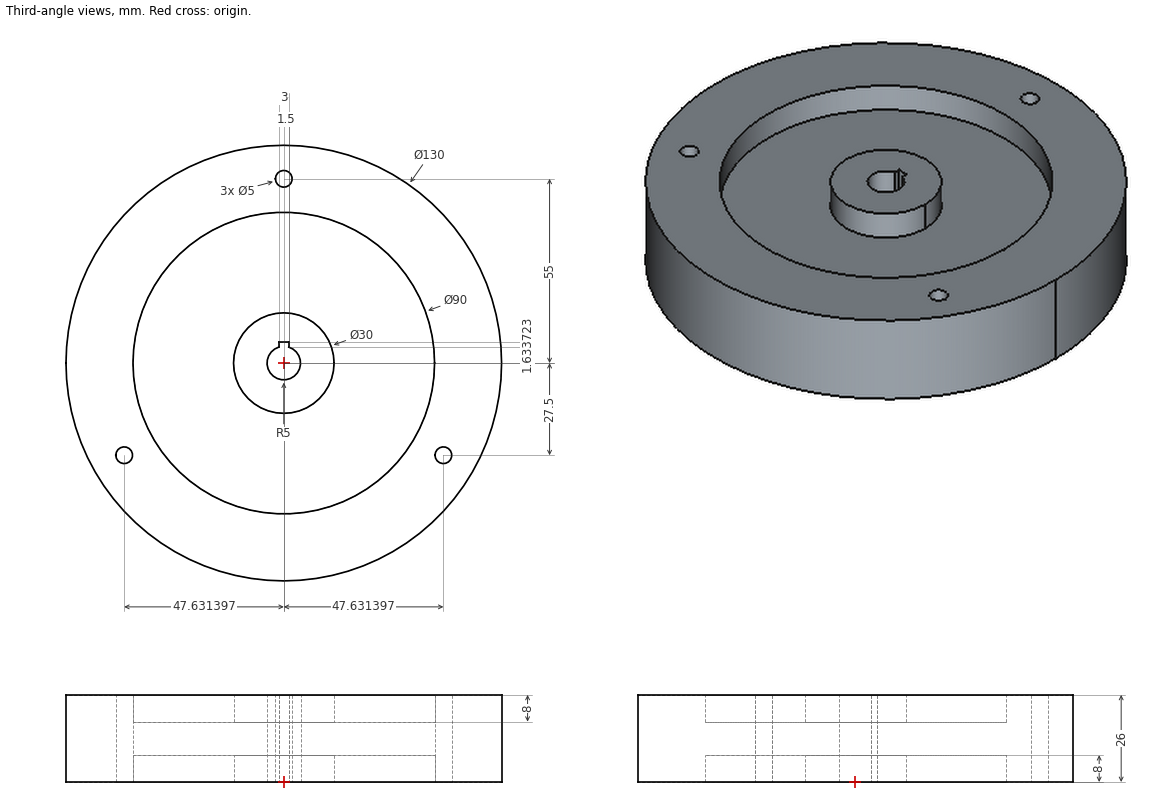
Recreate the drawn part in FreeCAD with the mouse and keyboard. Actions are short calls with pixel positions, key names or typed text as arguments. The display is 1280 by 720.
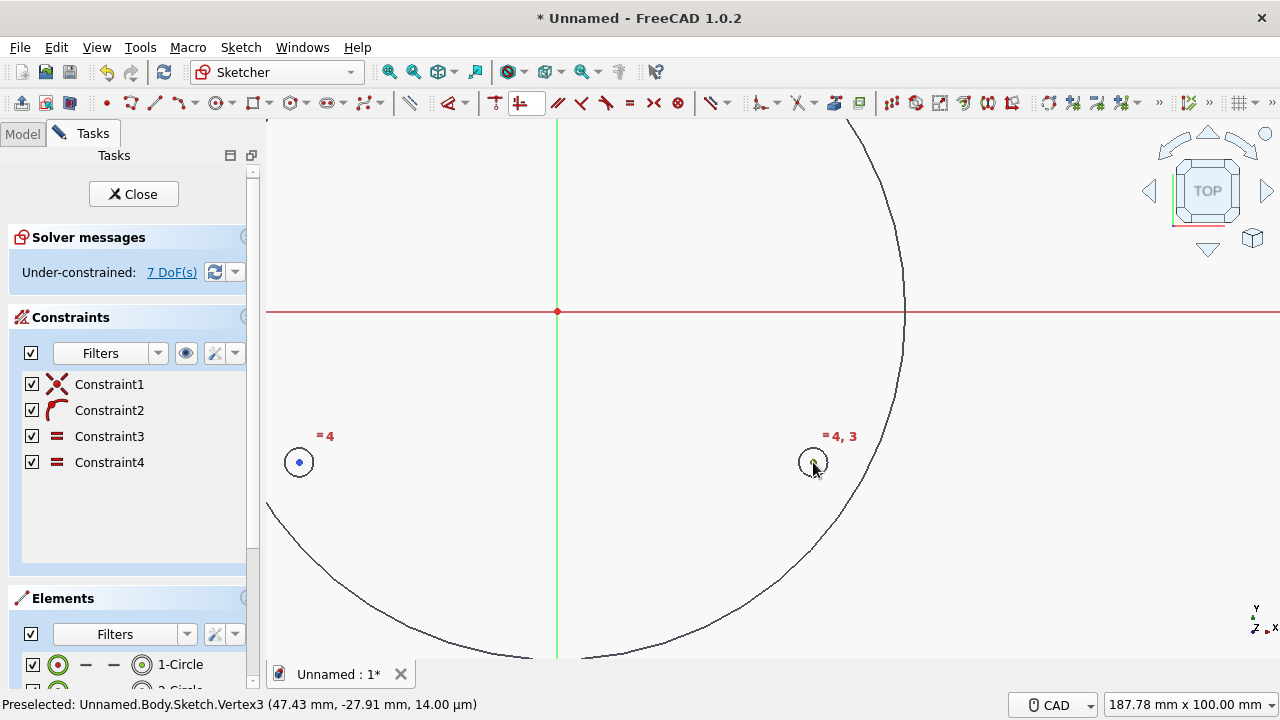
click(299, 462)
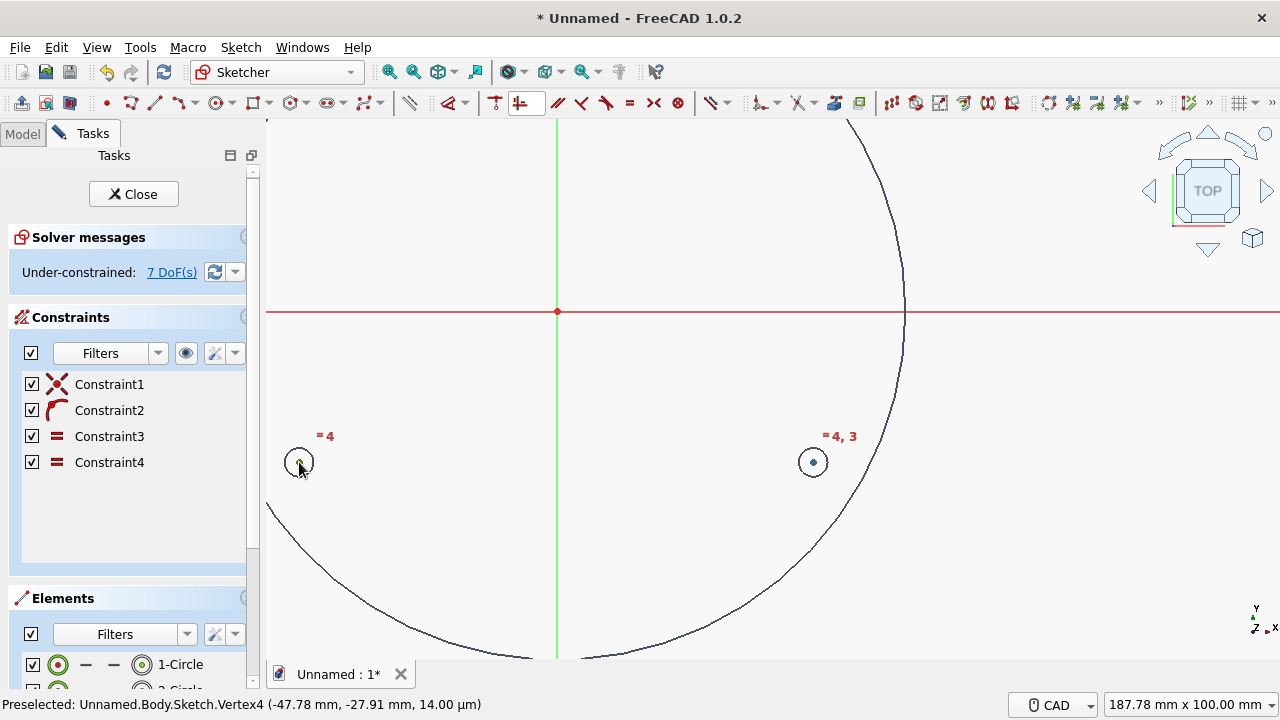
key(h)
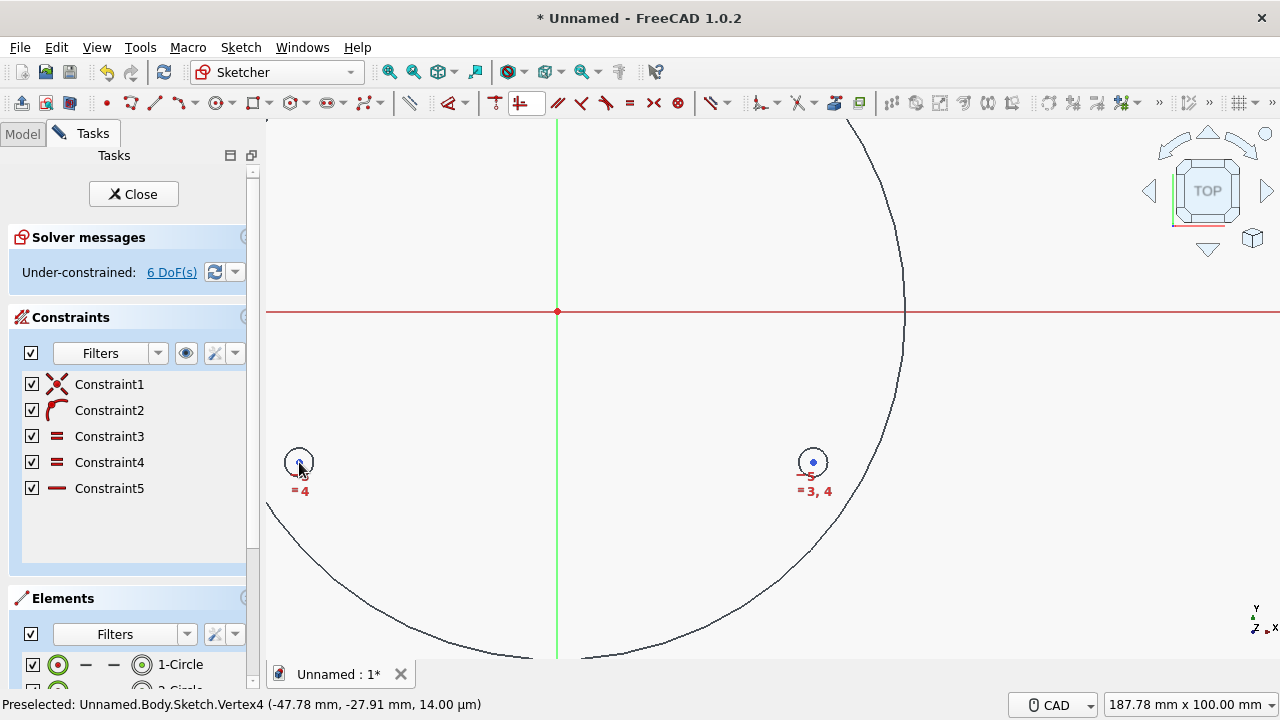
click(448, 104)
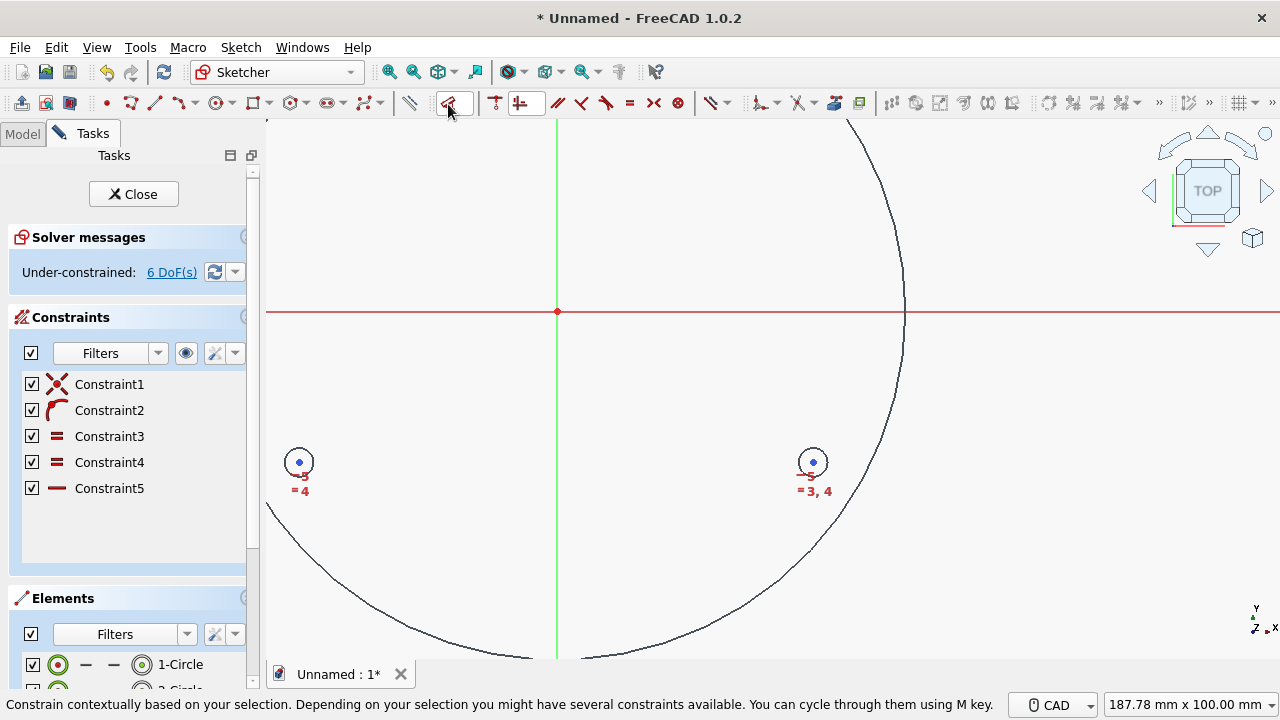
click(312, 559)
click(827, 579)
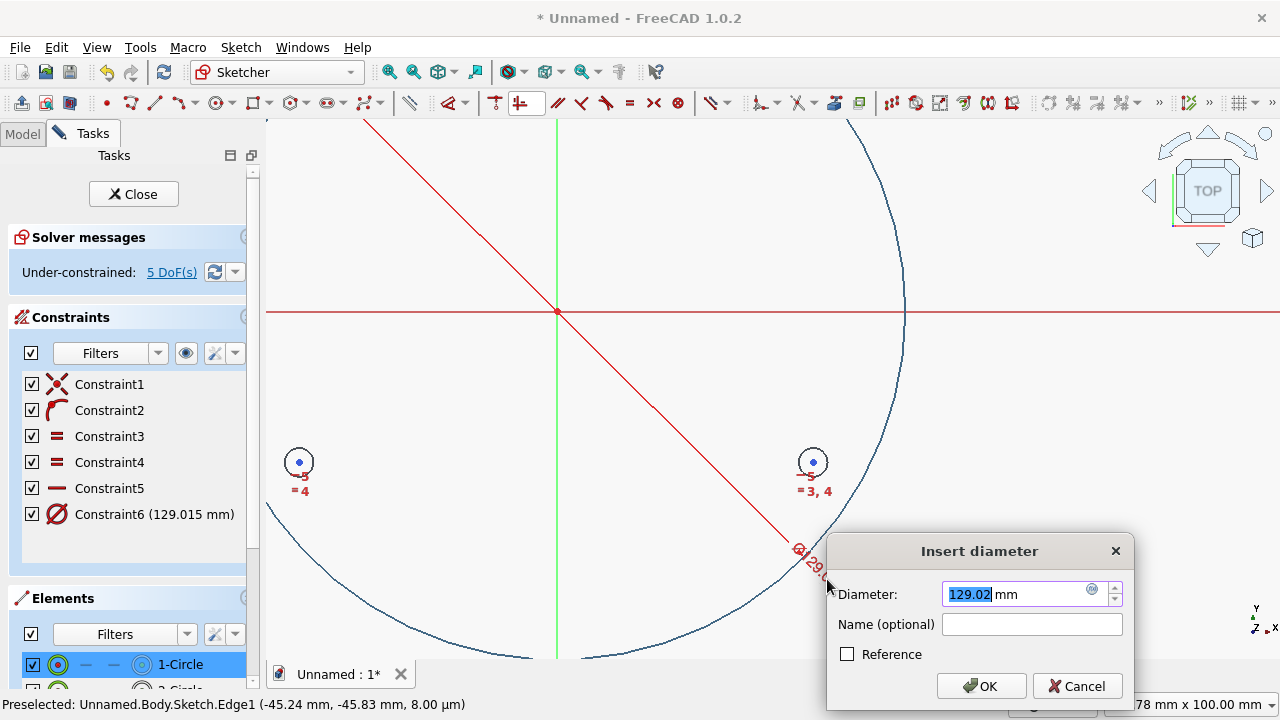
text(130)
key(Return)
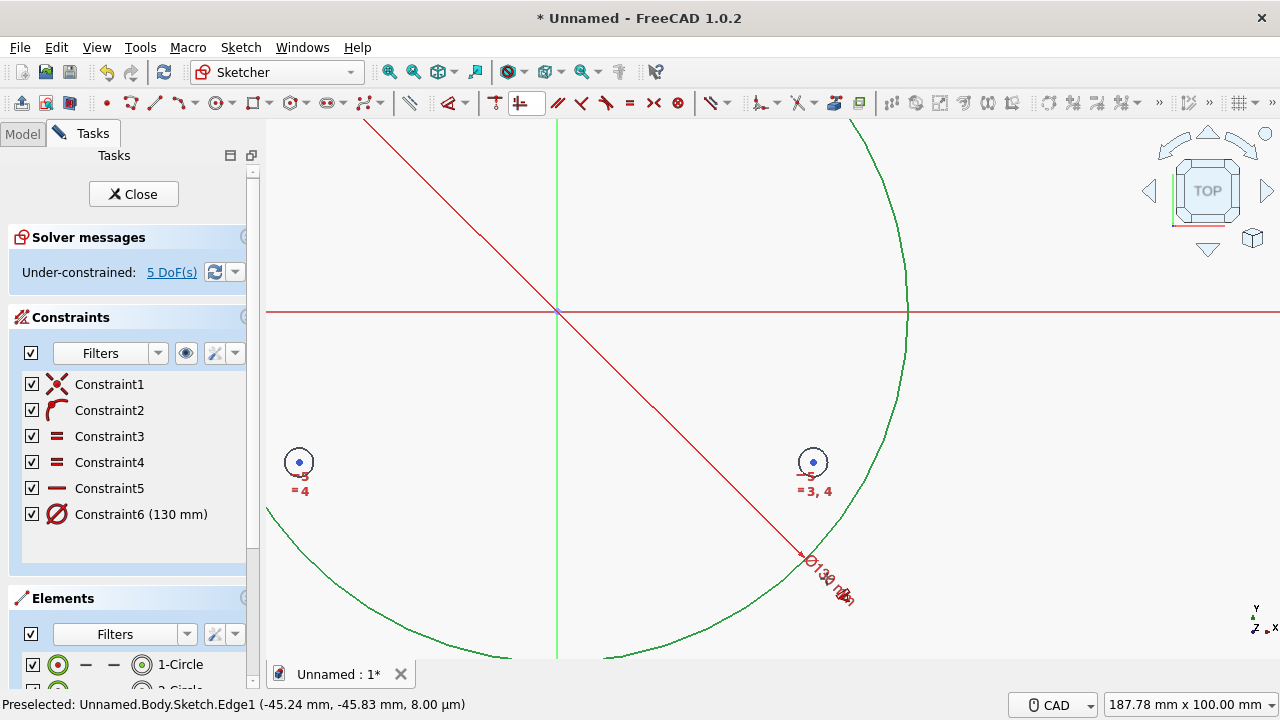
scroll(825, 452, down, 4)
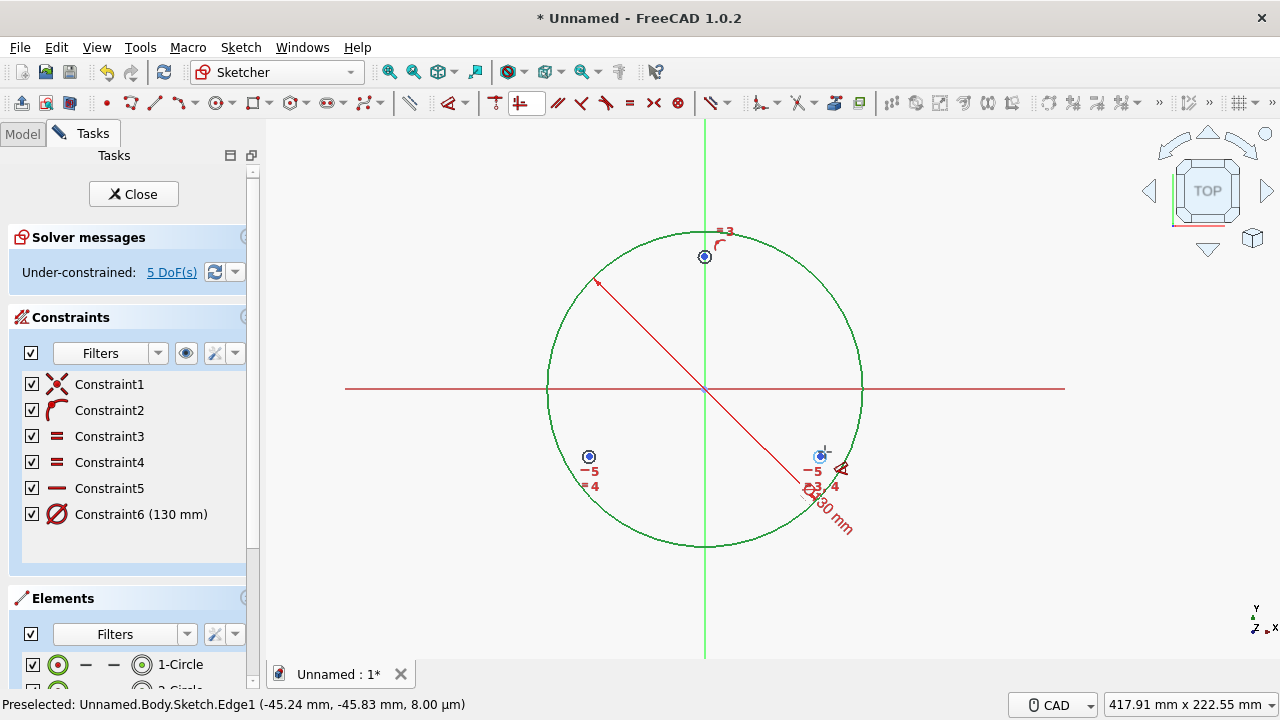
scroll(709, 252, up, 6)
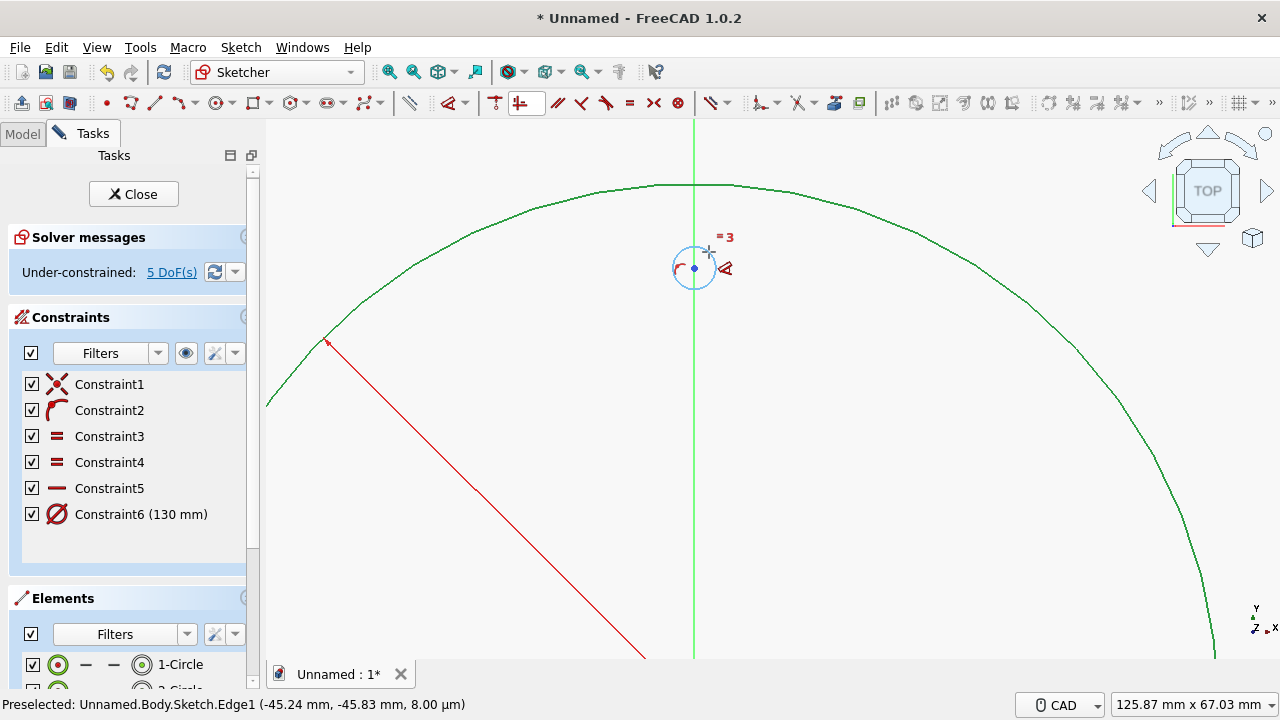
click(710, 253)
click(733, 231)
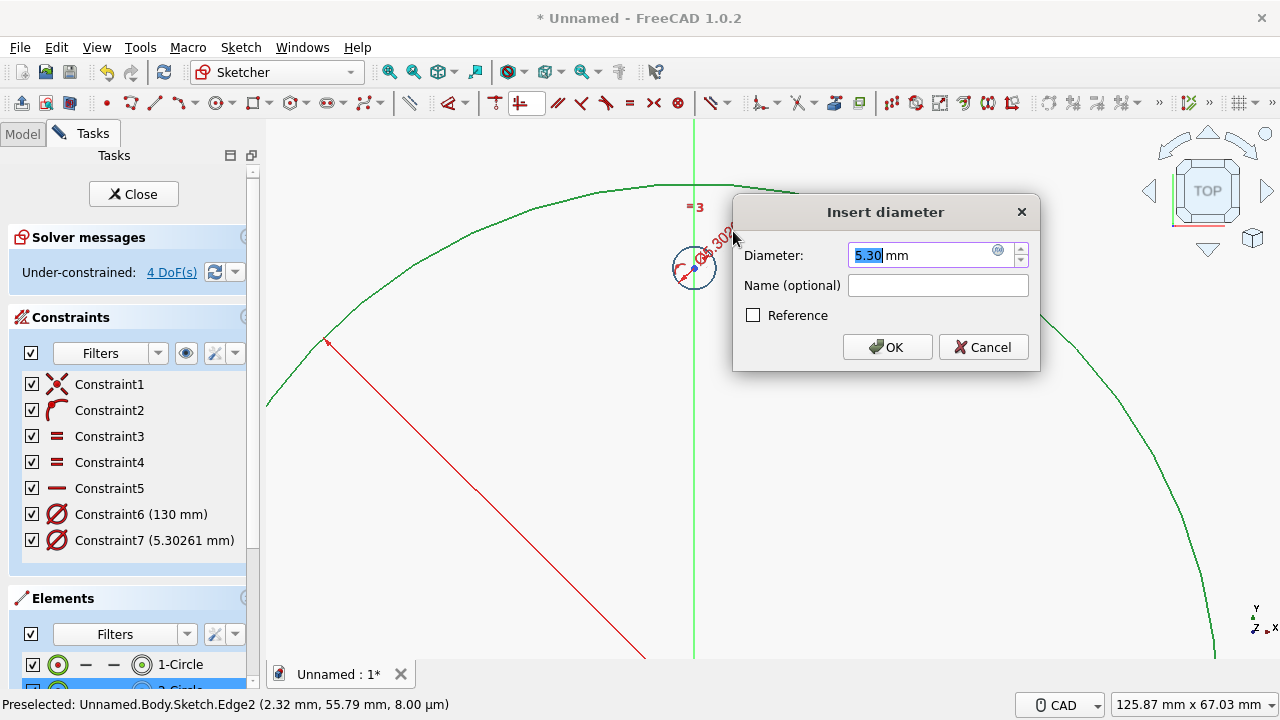
text(5)
key(Return)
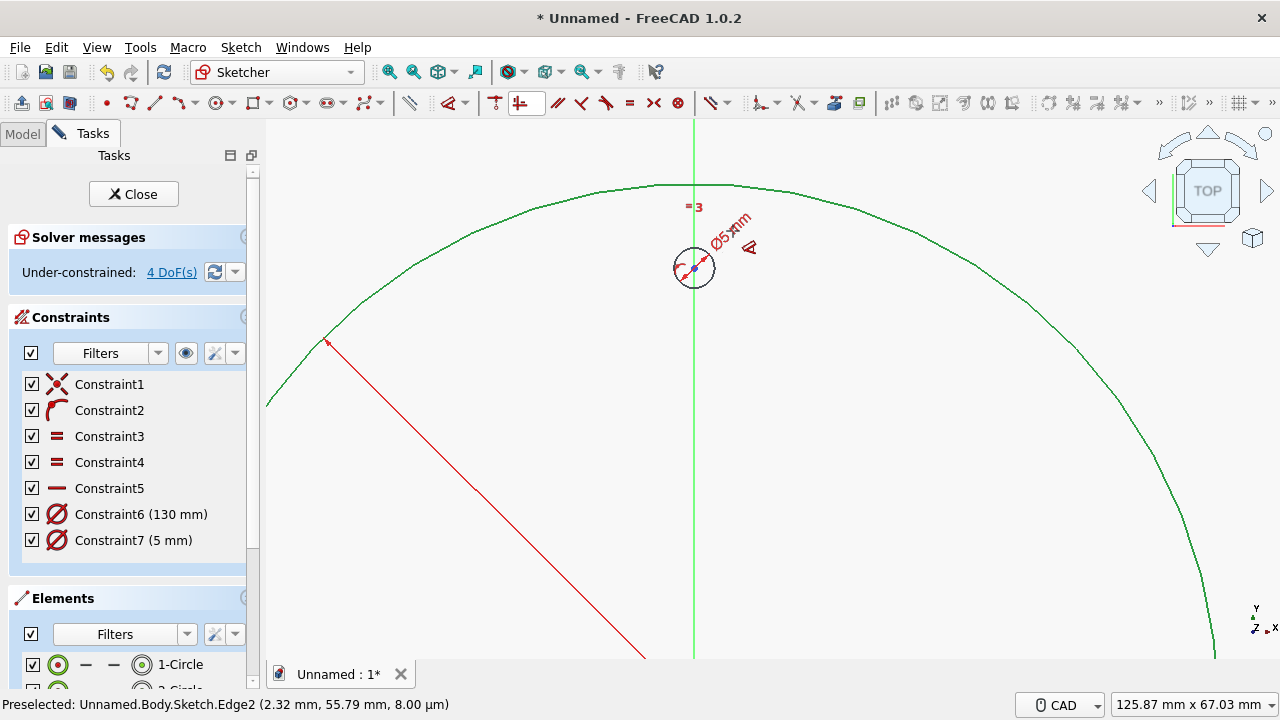
click(694, 268)
click(728, 450)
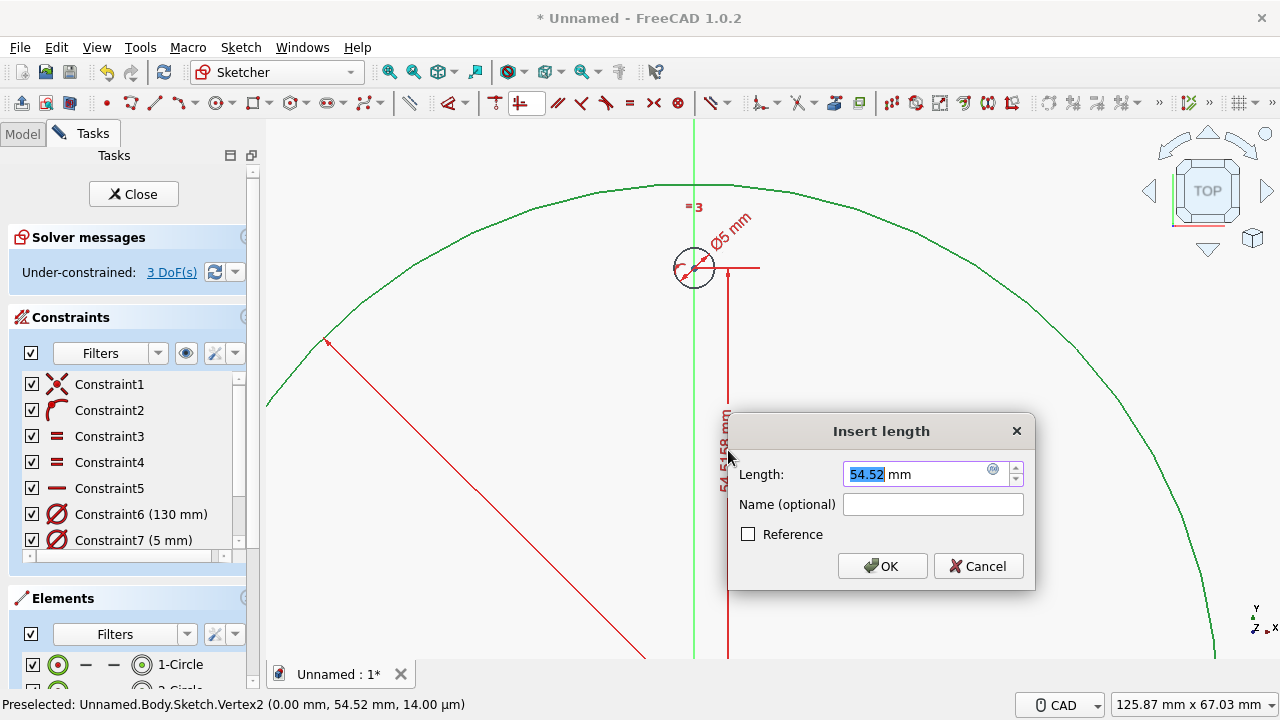
text(55)
key(Return)